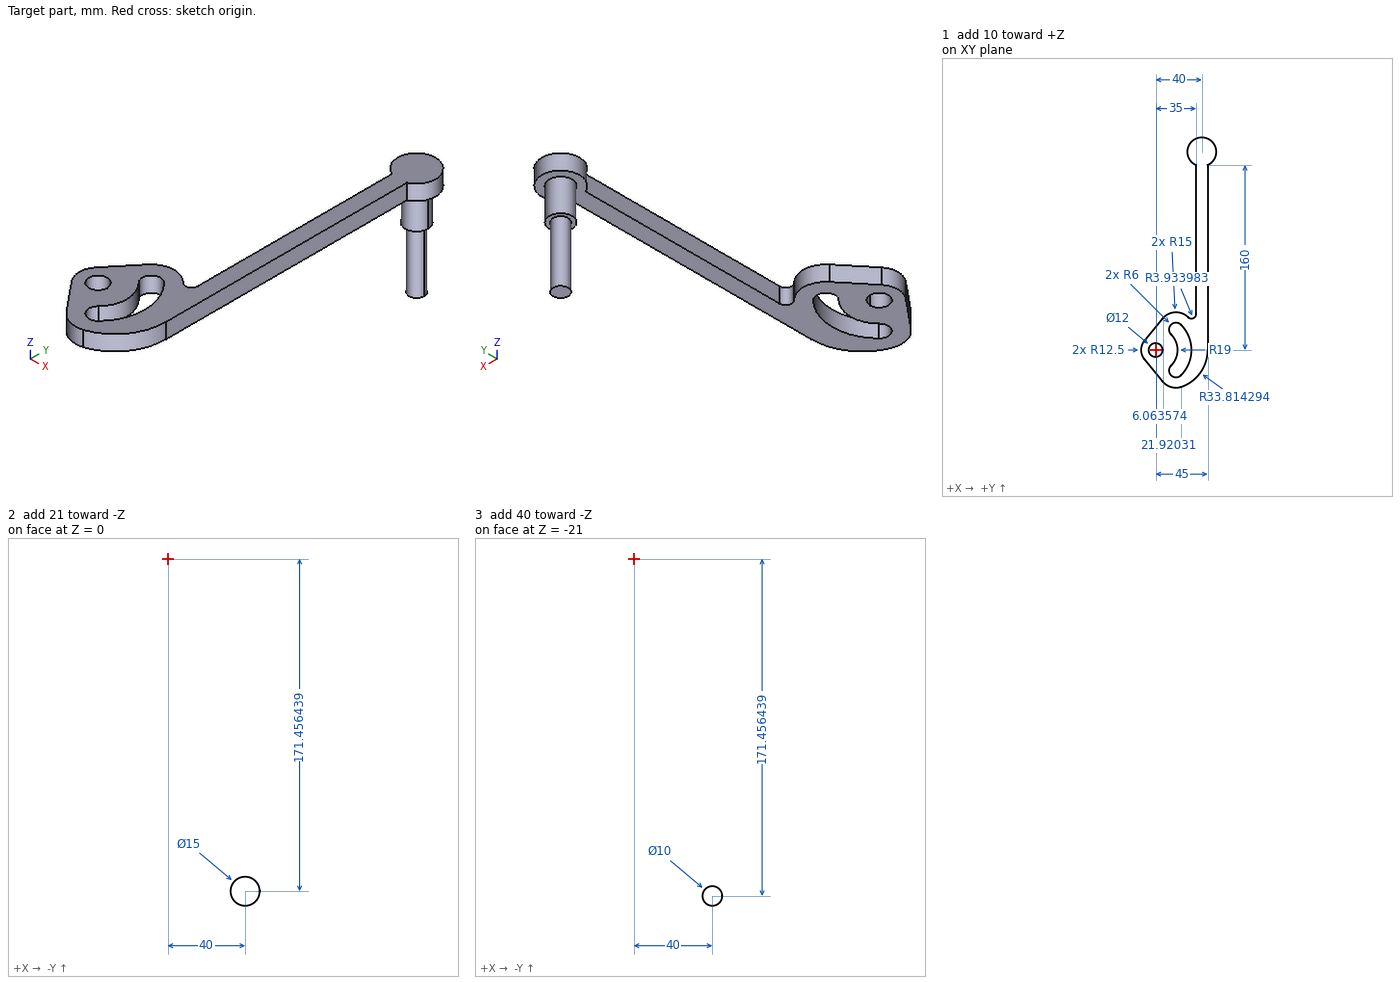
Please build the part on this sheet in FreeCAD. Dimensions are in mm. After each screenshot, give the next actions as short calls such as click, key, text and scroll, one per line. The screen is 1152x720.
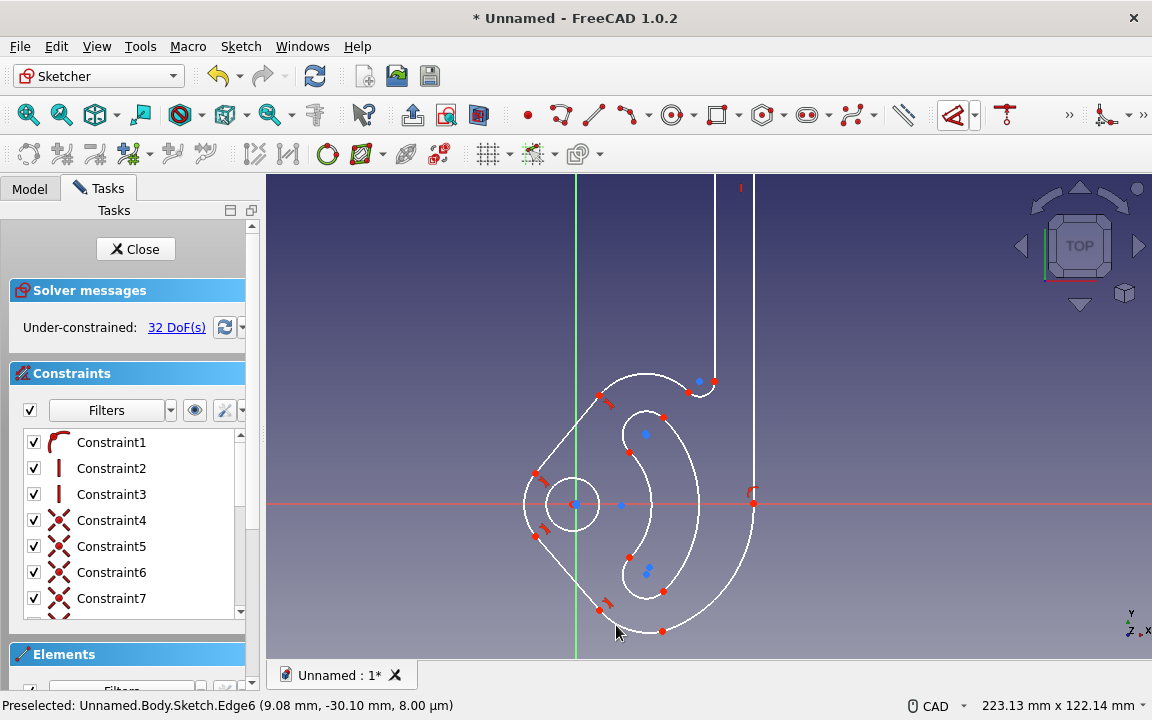
click(715, 228)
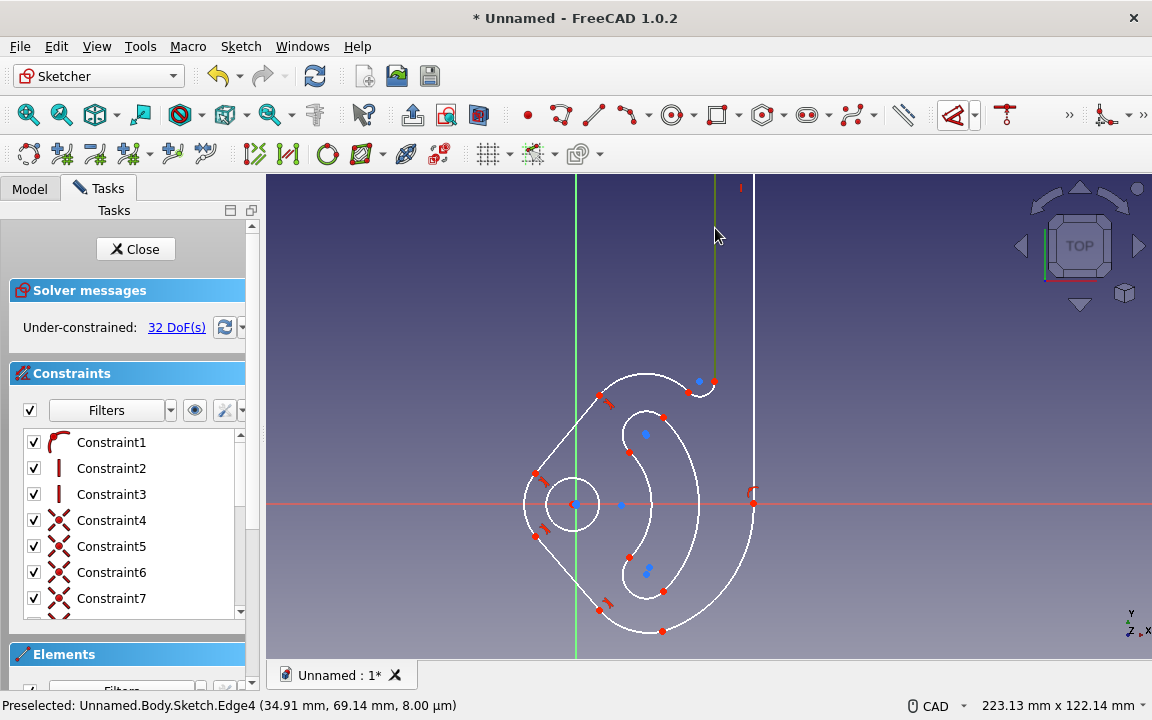
scroll(698, 397, up, 2)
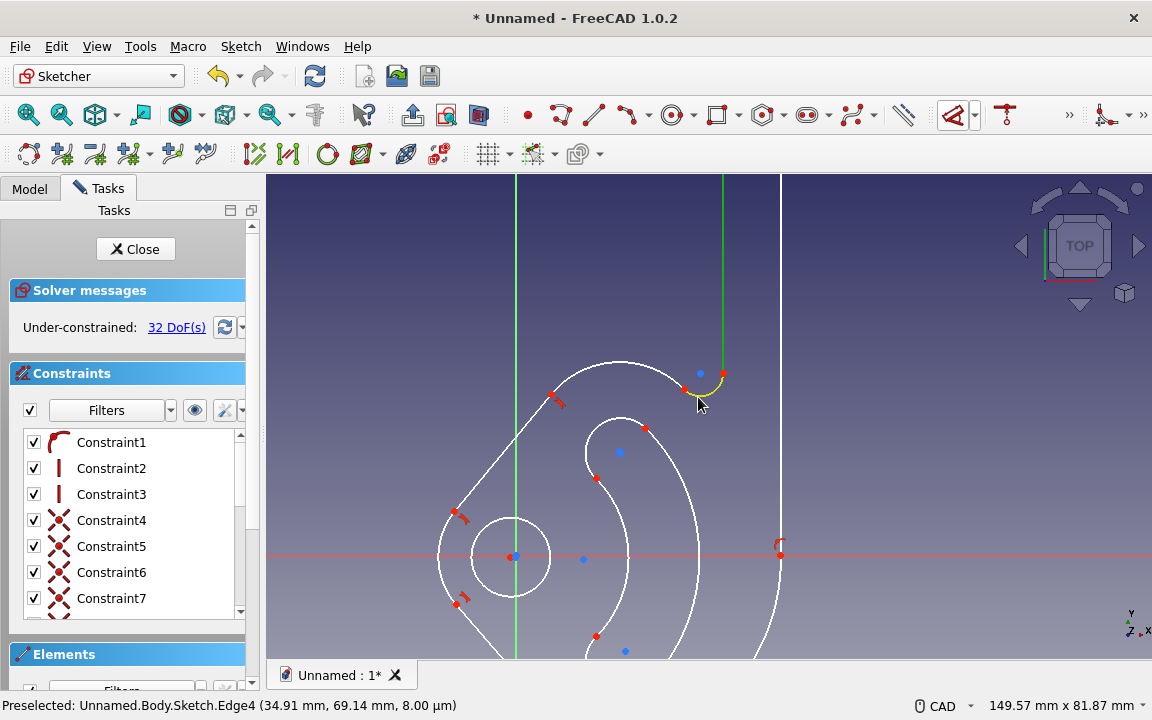
click(698, 396)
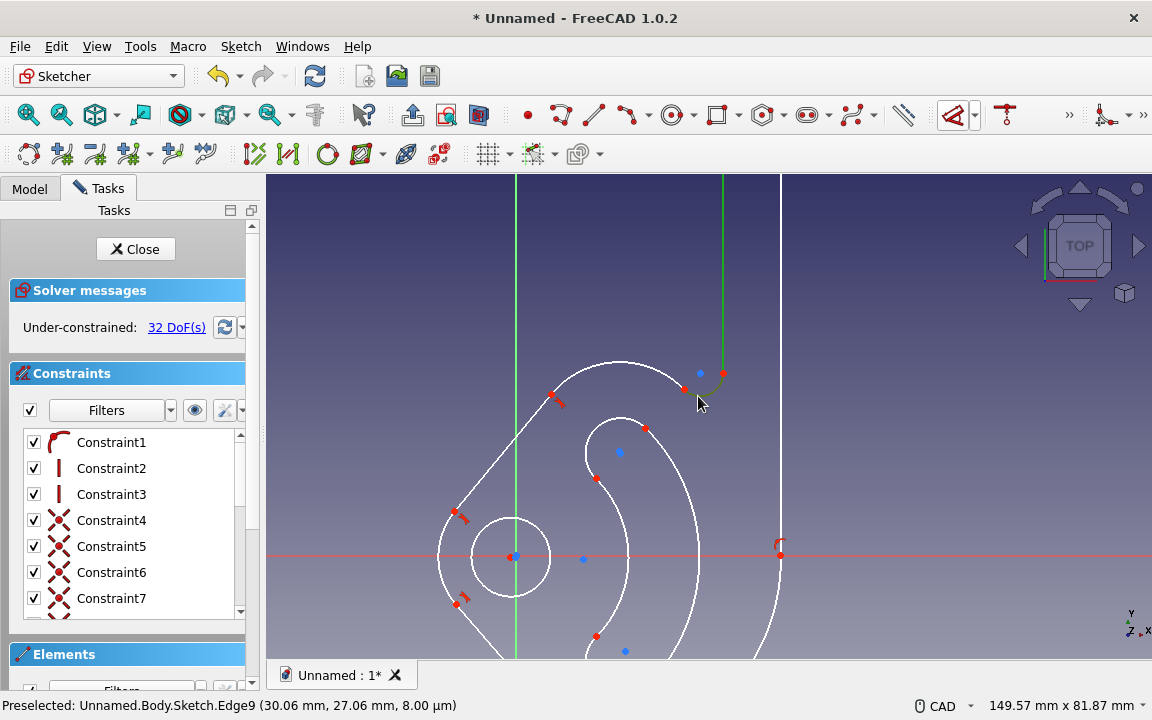
key(t)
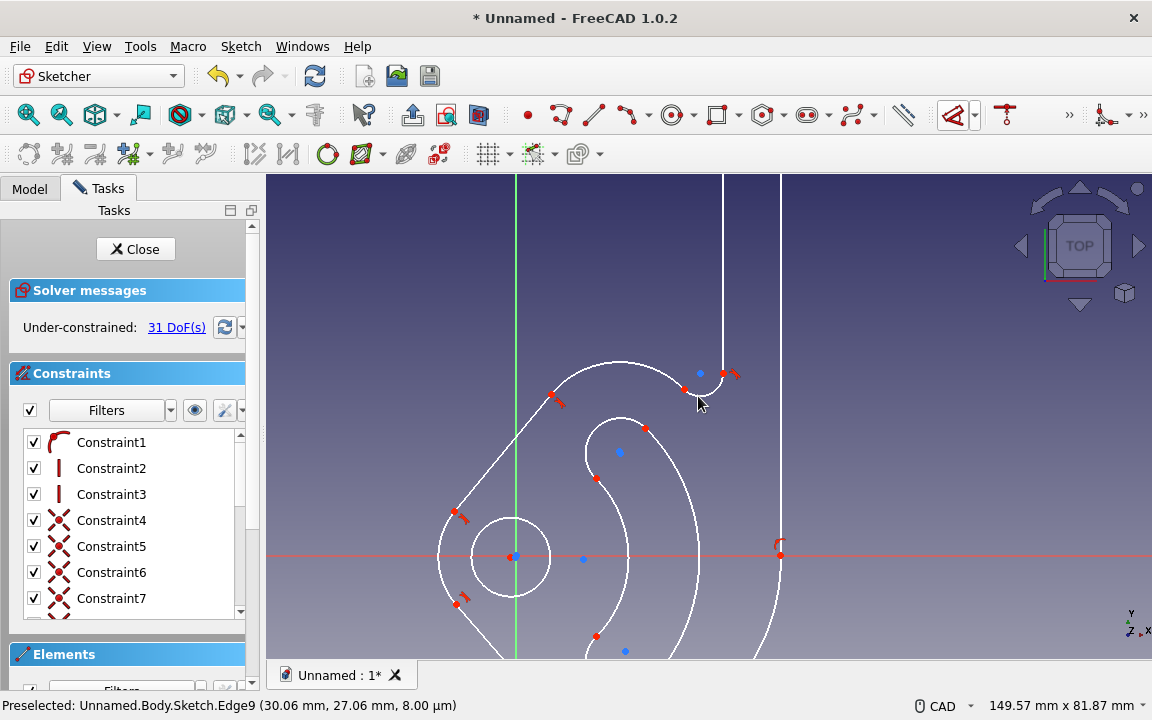
click(699, 396)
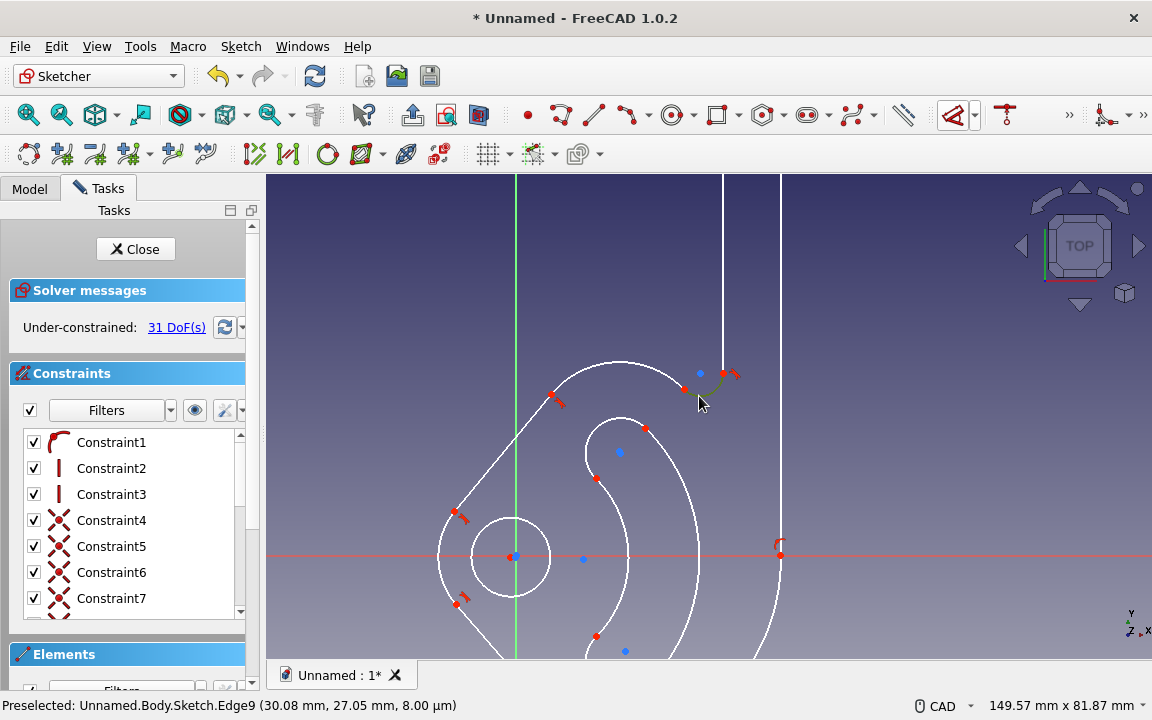
scroll(650, 518, down, 7)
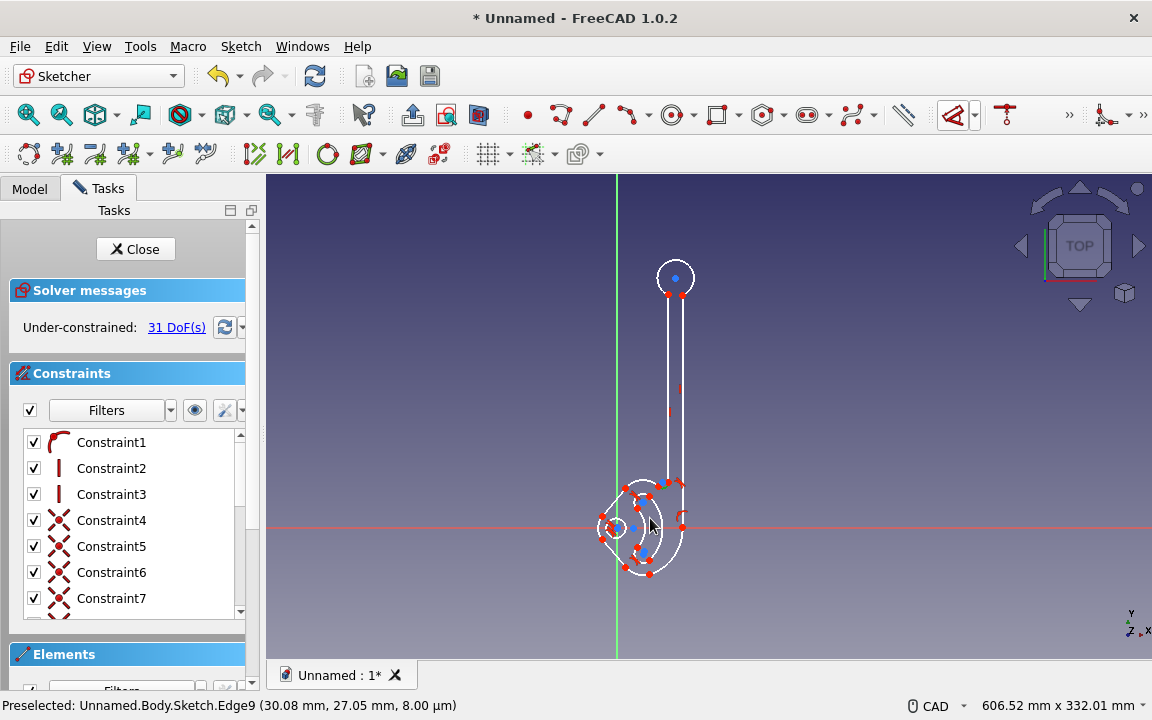
scroll(649, 481, up, 2)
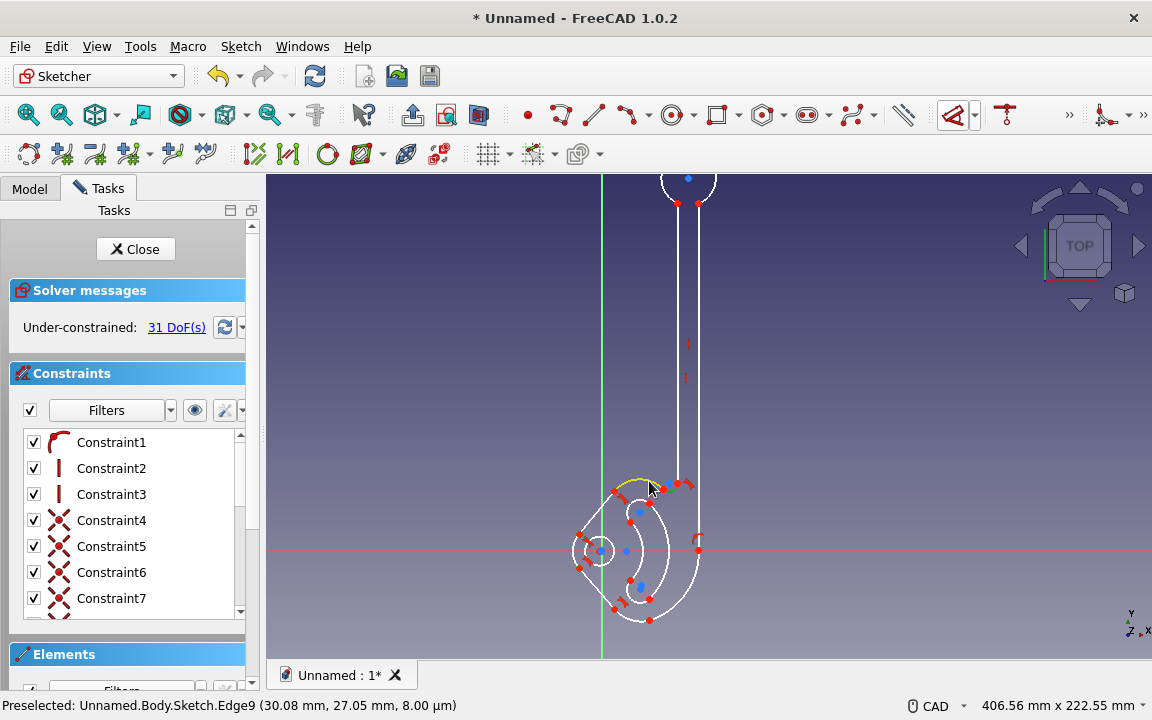
click(649, 481)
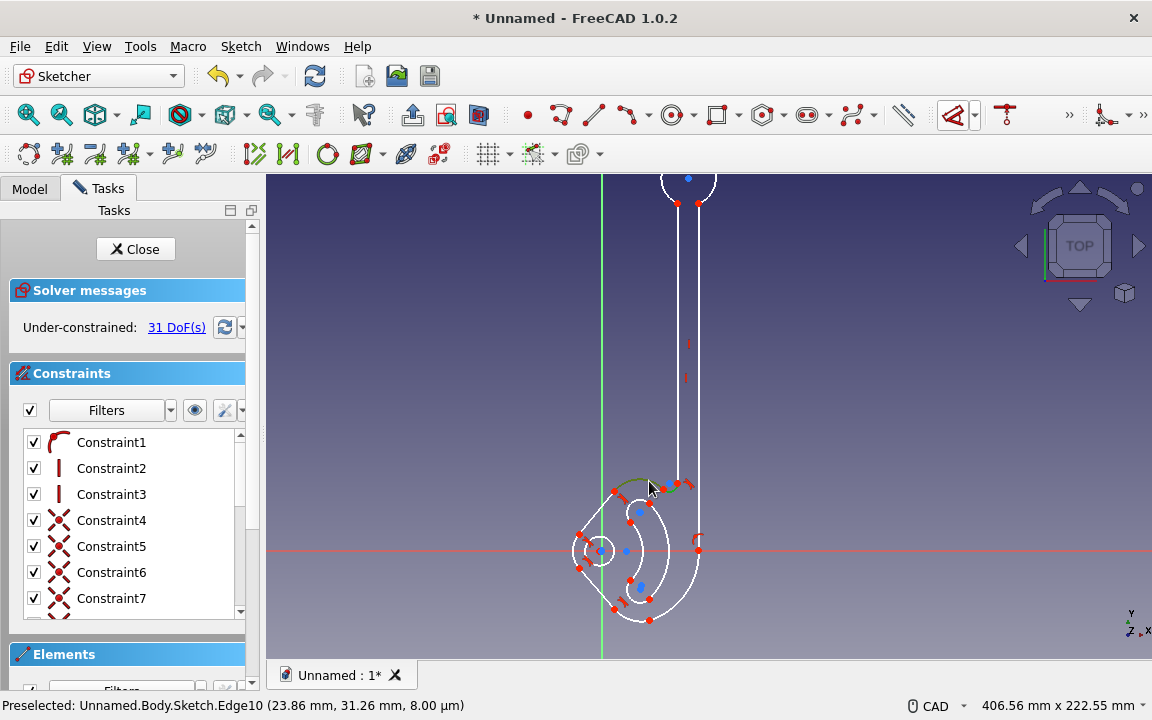
key(t)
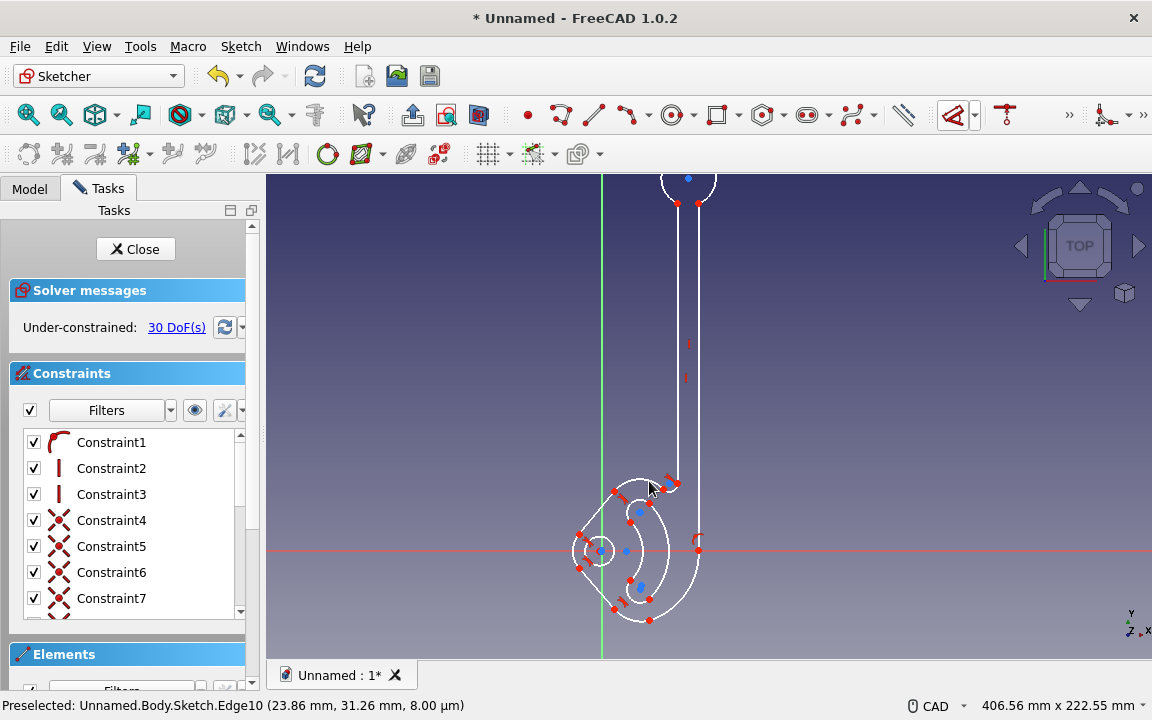
click(641, 564)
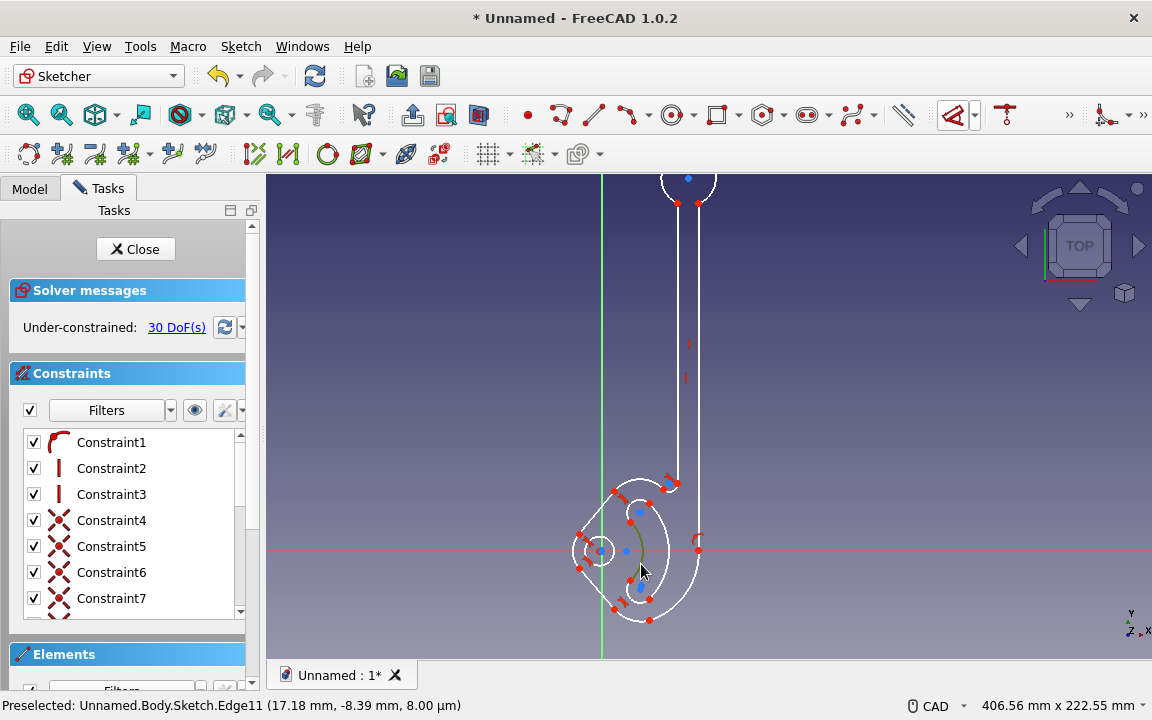
click(638, 500)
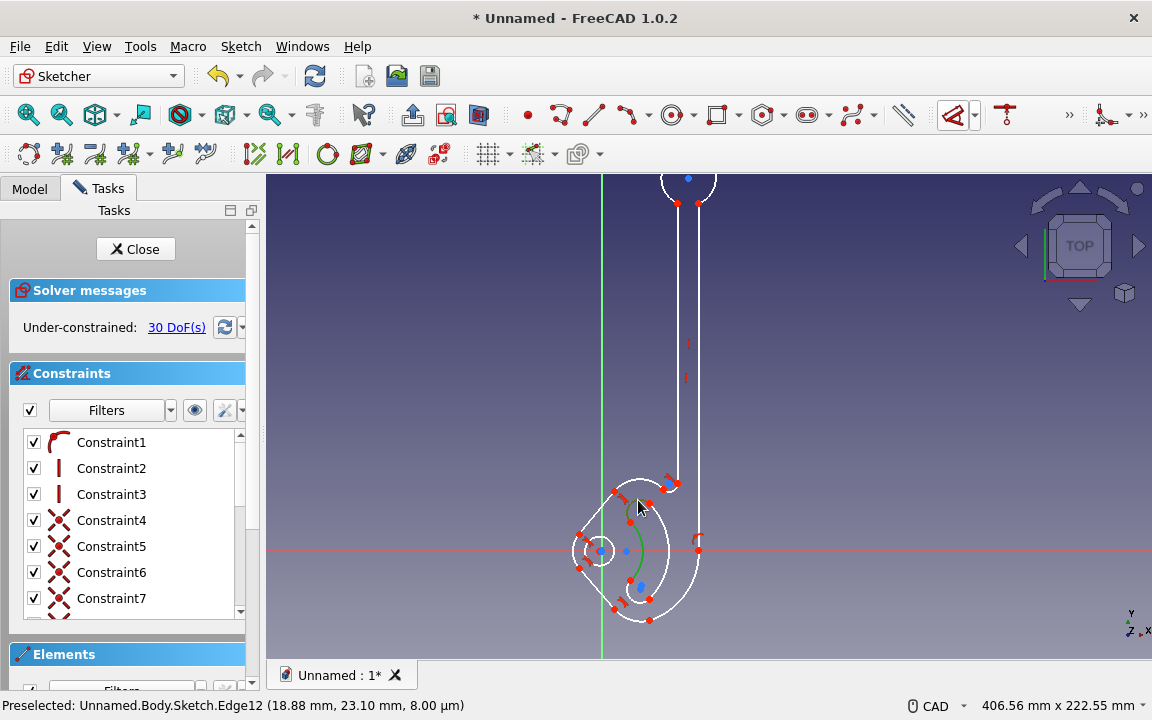
key(t)